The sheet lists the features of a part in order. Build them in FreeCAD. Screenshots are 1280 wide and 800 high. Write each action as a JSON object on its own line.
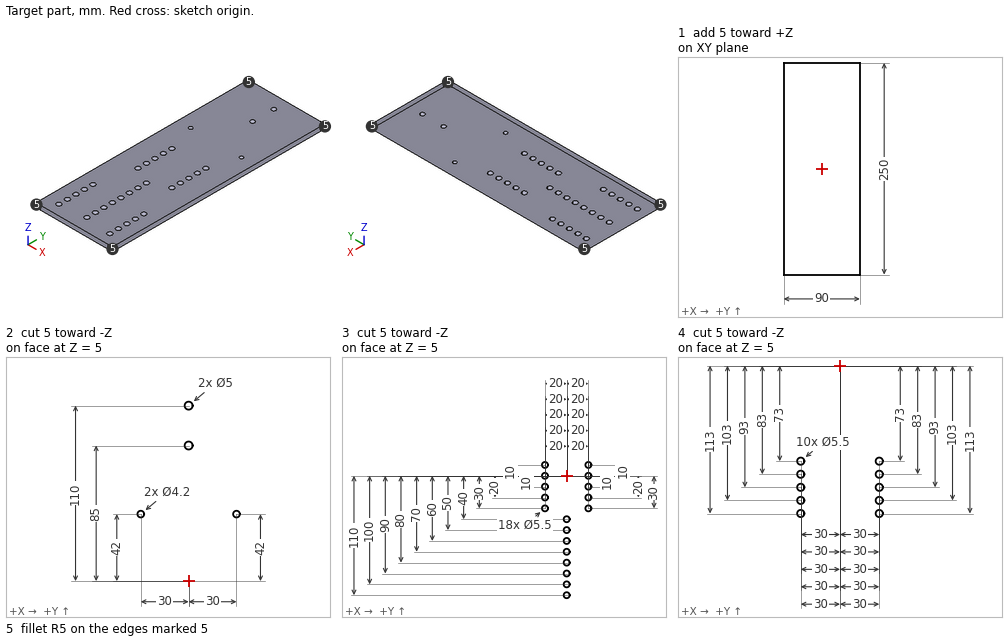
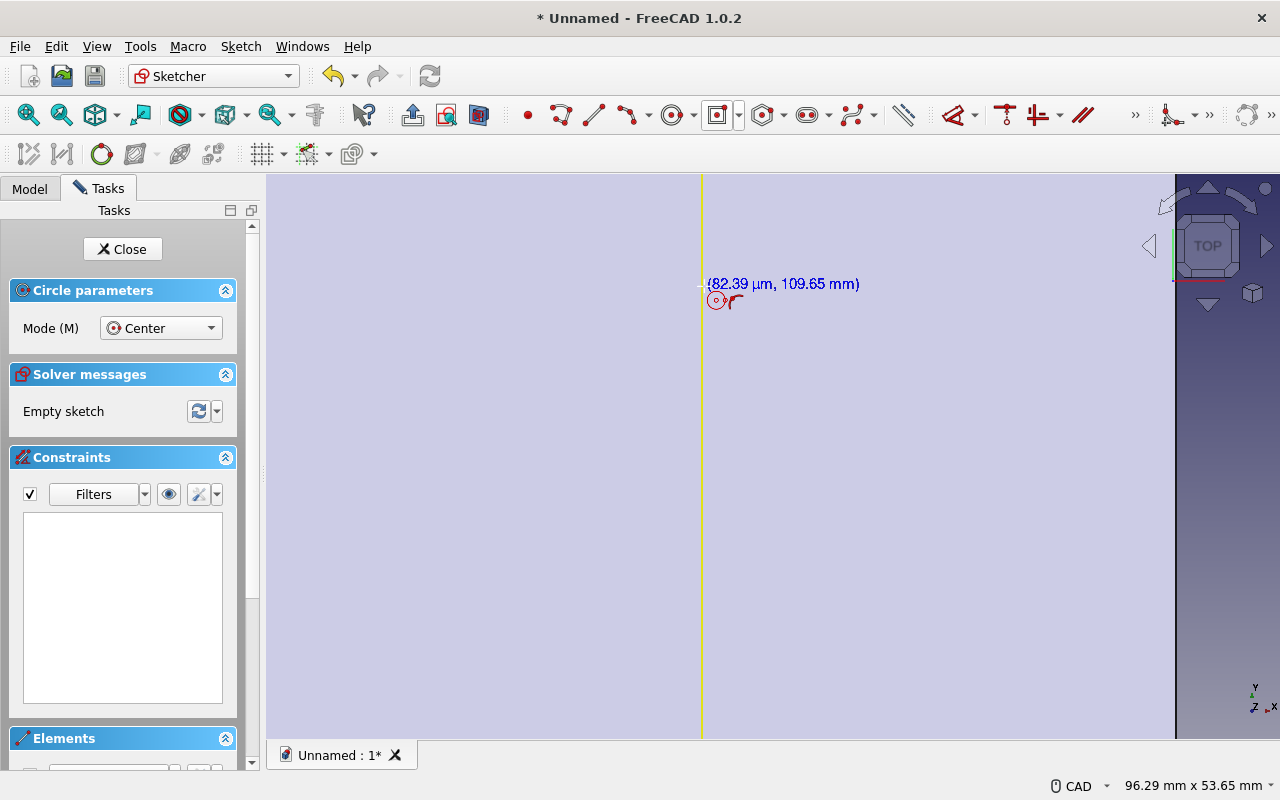
{"action": "left_click", "coordinate": [702, 285]}
{"action": "mouse_move", "coordinate": [721, 267]}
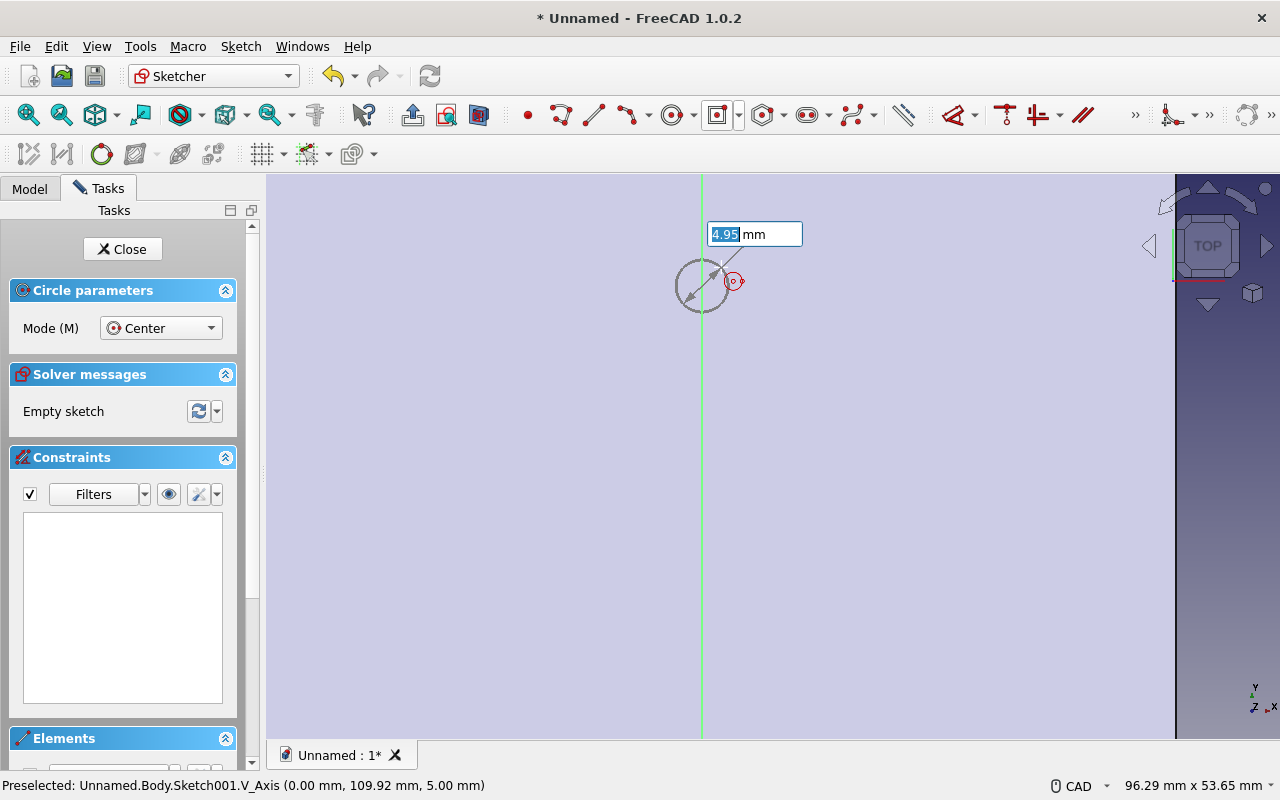
{"action": "type", "text": "5"}
{"action": "key", "text": "Return"}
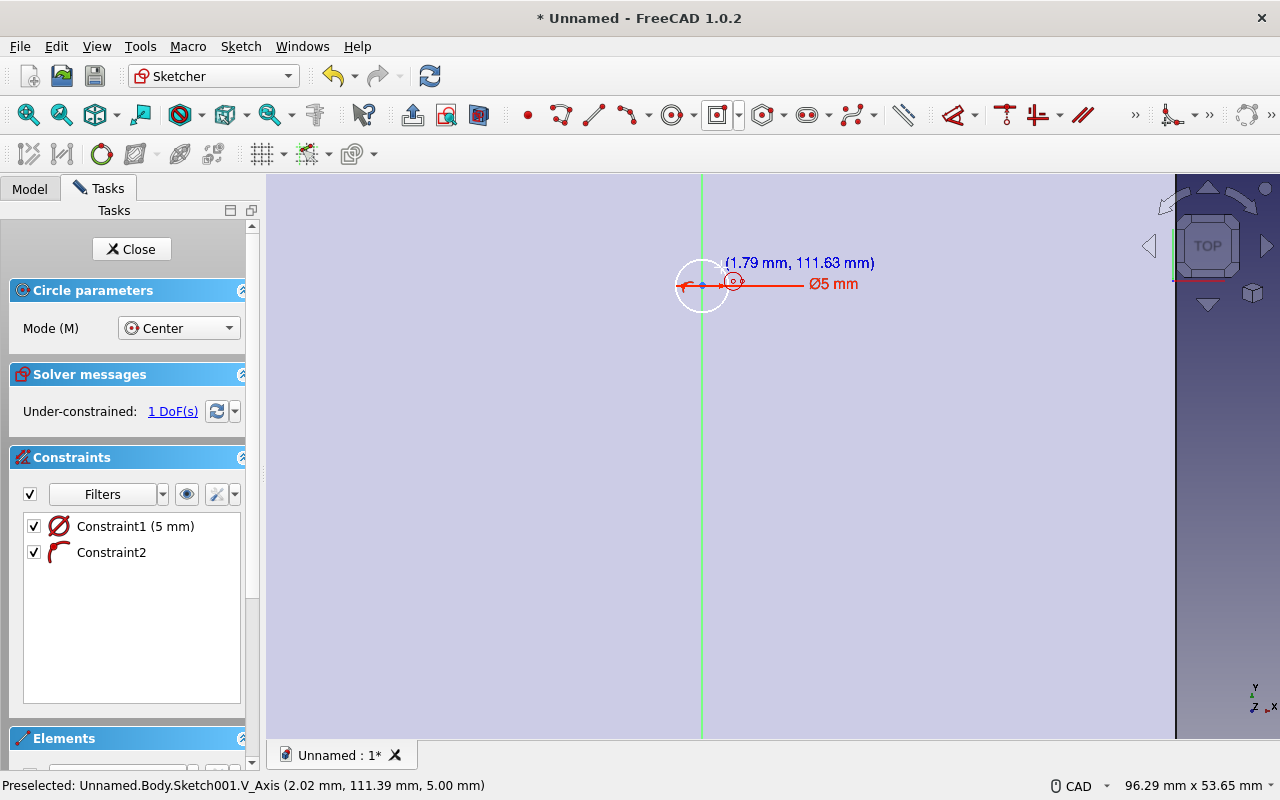
{"action": "left_click", "coordinate": [702, 548]}
{"action": "mouse_move", "coordinate": [721, 530]}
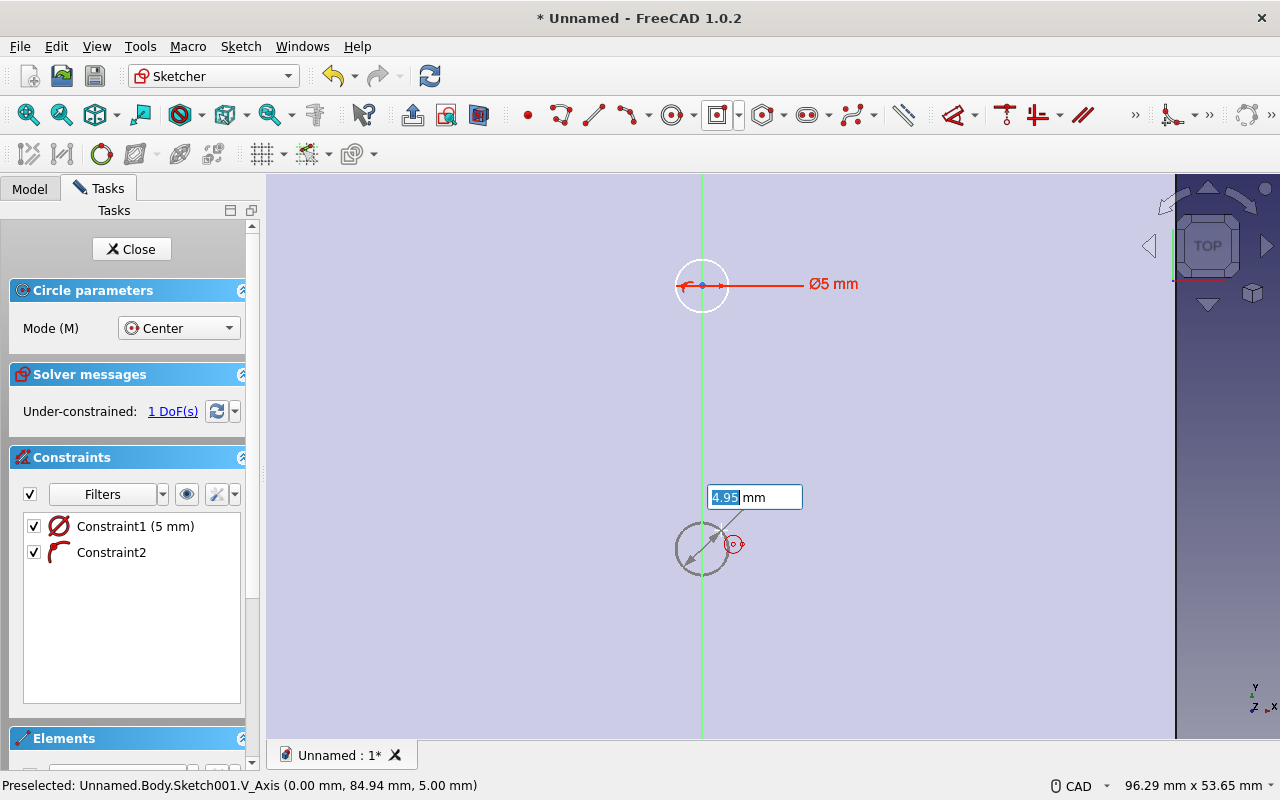
{"action": "type", "text": "5"}
{"action": "key", "text": "Return"}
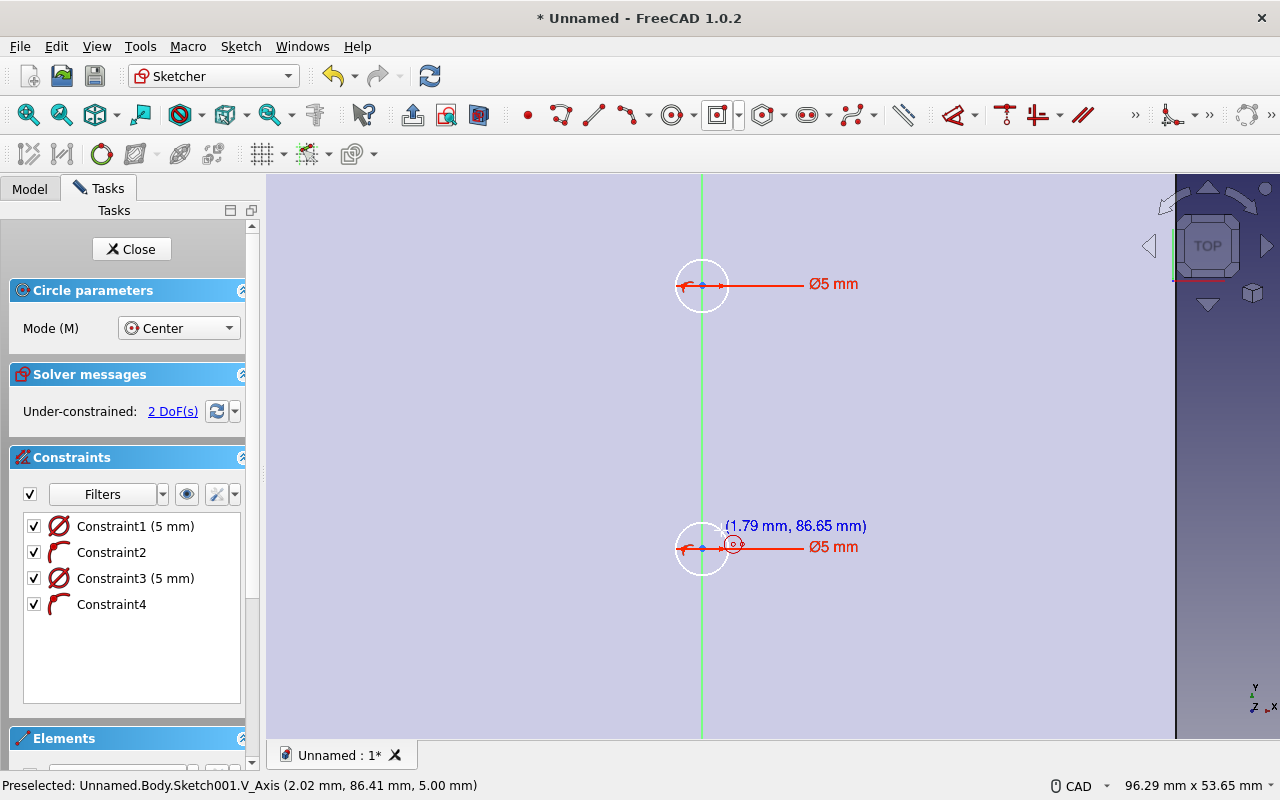
{"action": "scroll", "coordinate": [706, 286], "scroll_direction": "down", "scroll_amount": 6}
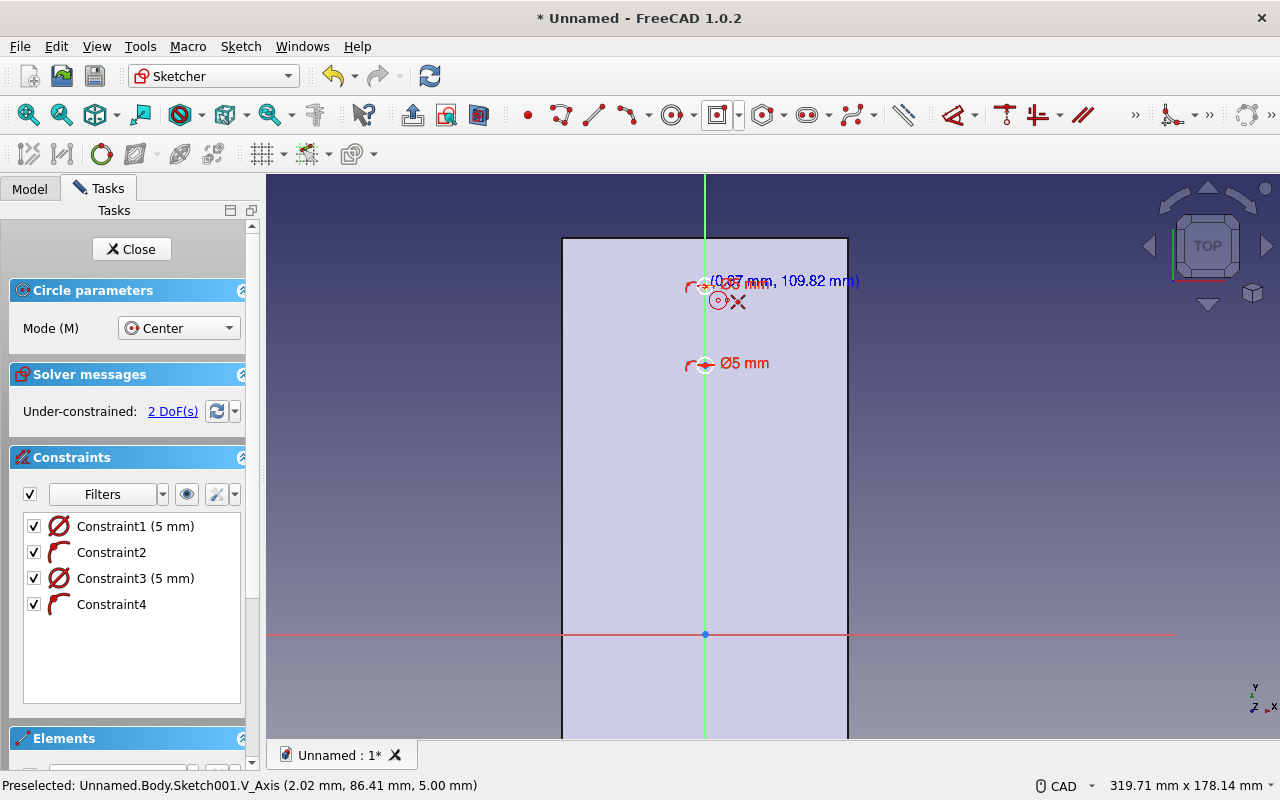
{"action": "scroll", "coordinate": [610, 502], "scroll_direction": "up", "scroll_amount": 7}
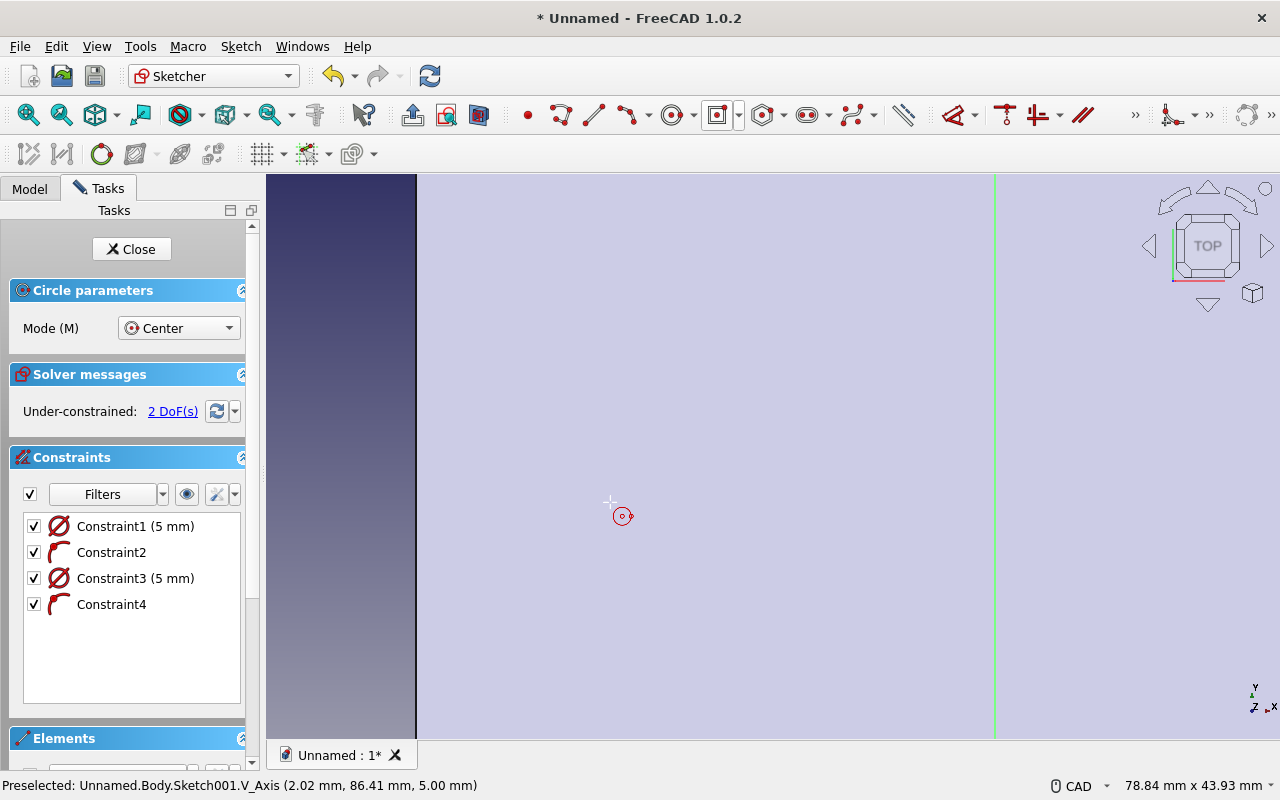
{"action": "scroll", "coordinate": [609, 503], "scroll_direction": "down", "scroll_amount": 7}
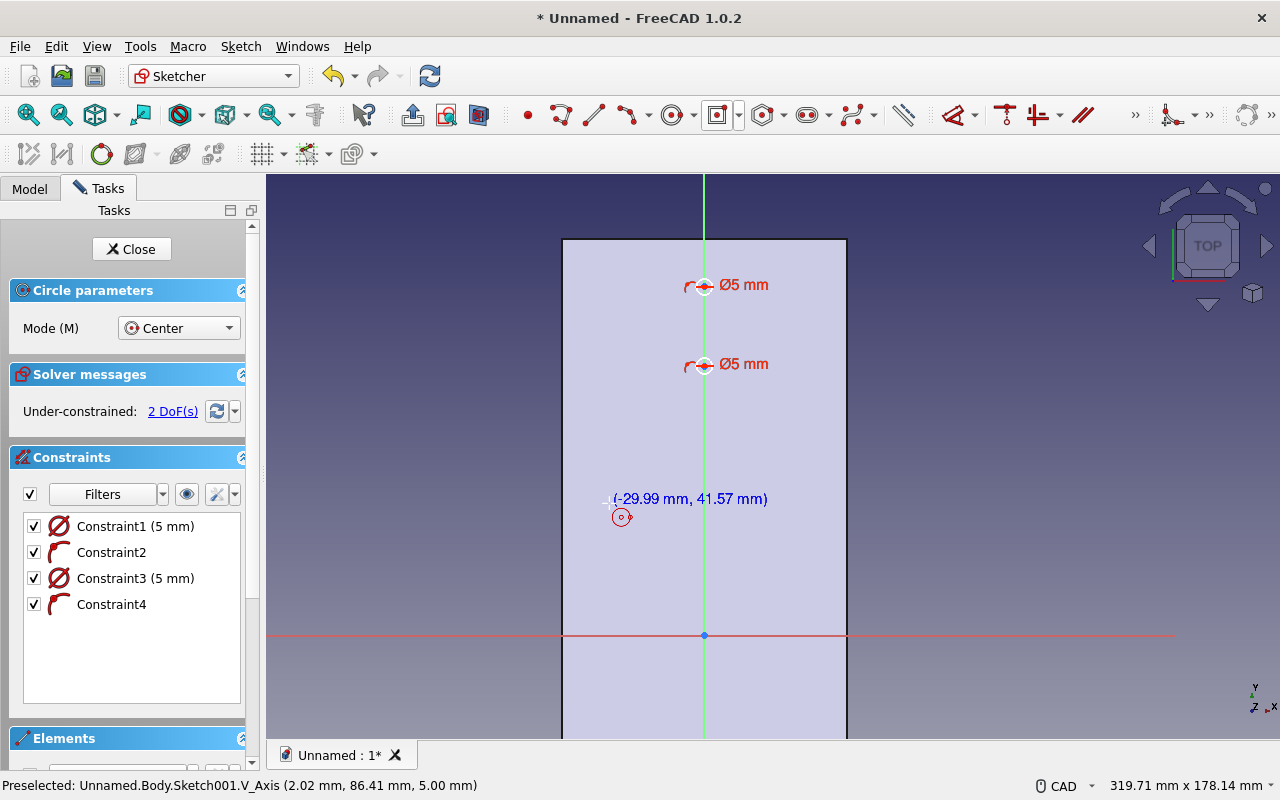
{"action": "left_click", "coordinate": [609, 502]}
{"action": "mouse_move", "coordinate": [614, 498]}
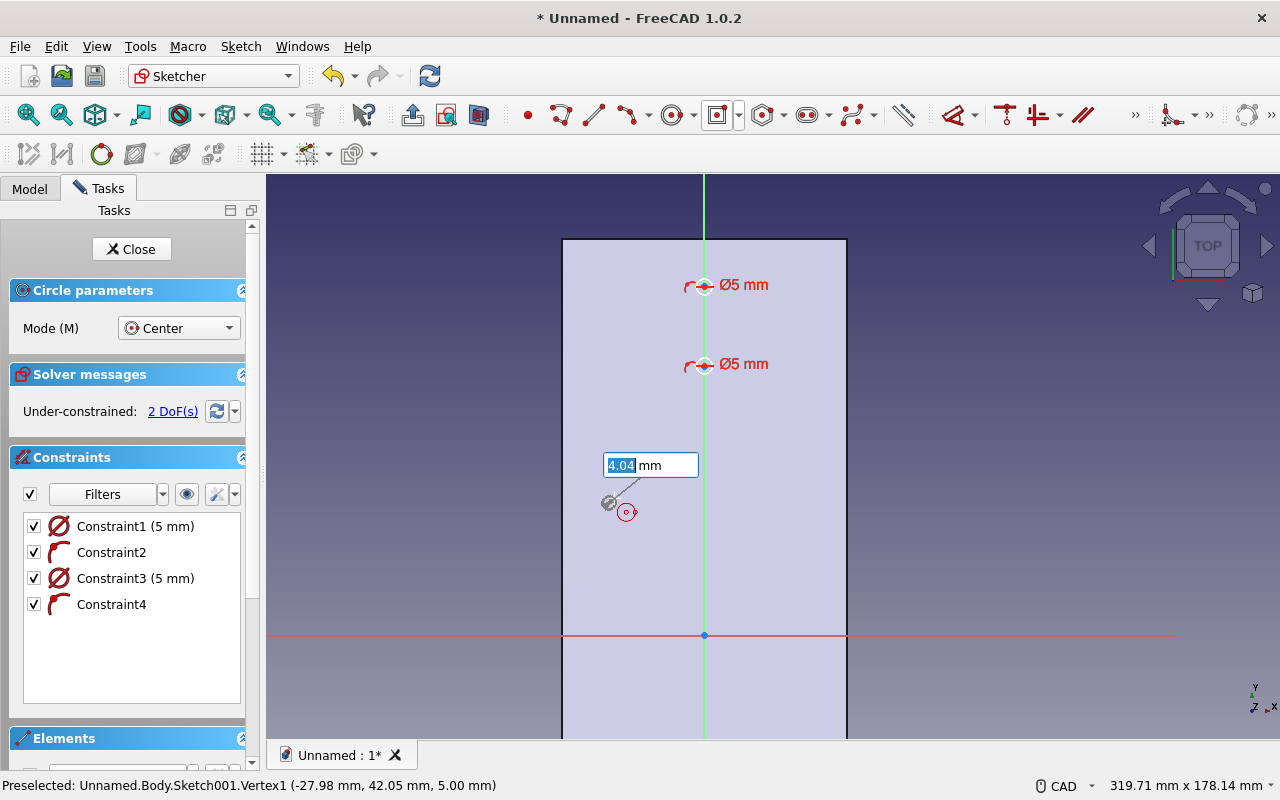
{"action": "type", "text": "4.2"}
{"action": "key", "text": "Return"}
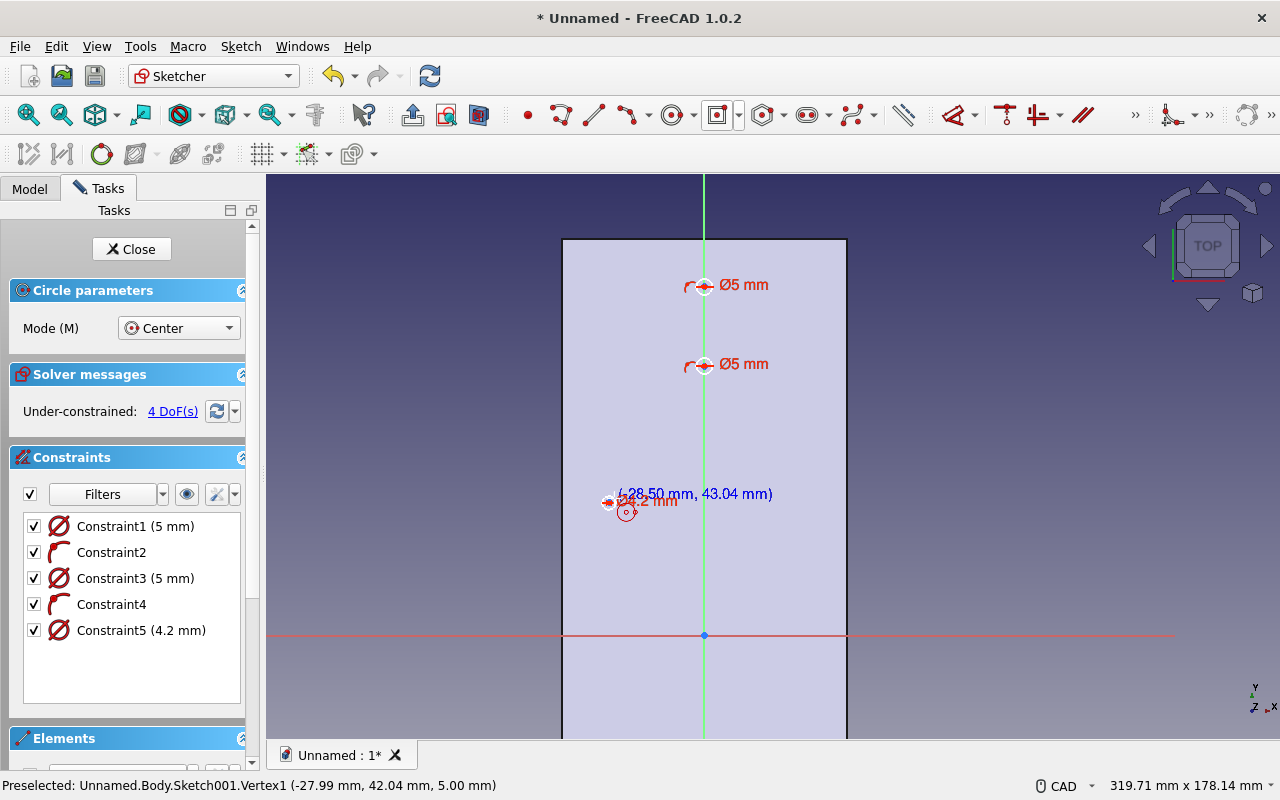
{"action": "scroll", "coordinate": [800, 502], "scroll_direction": "up", "scroll_amount": 7}